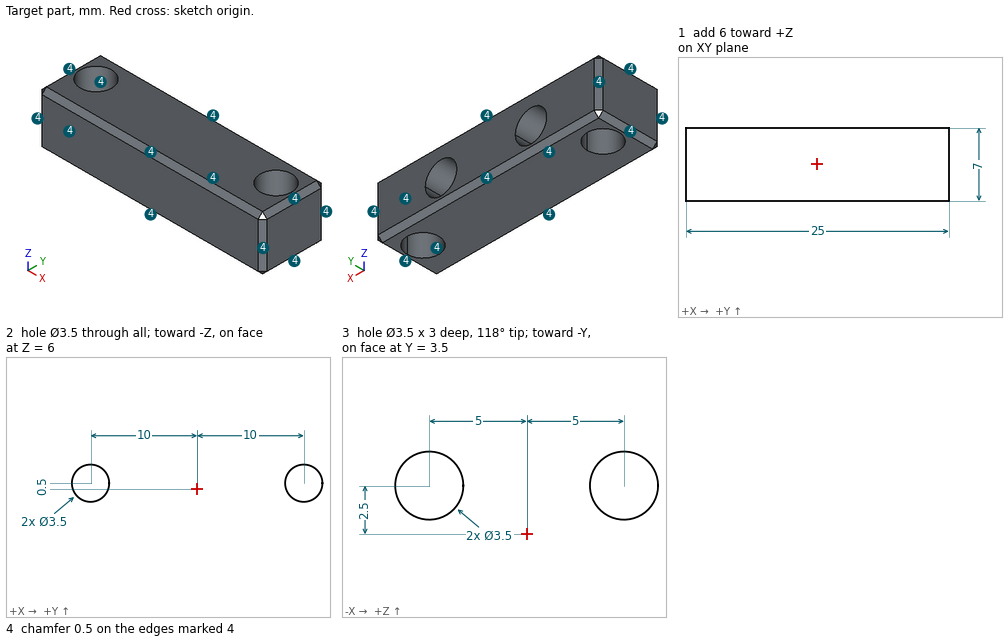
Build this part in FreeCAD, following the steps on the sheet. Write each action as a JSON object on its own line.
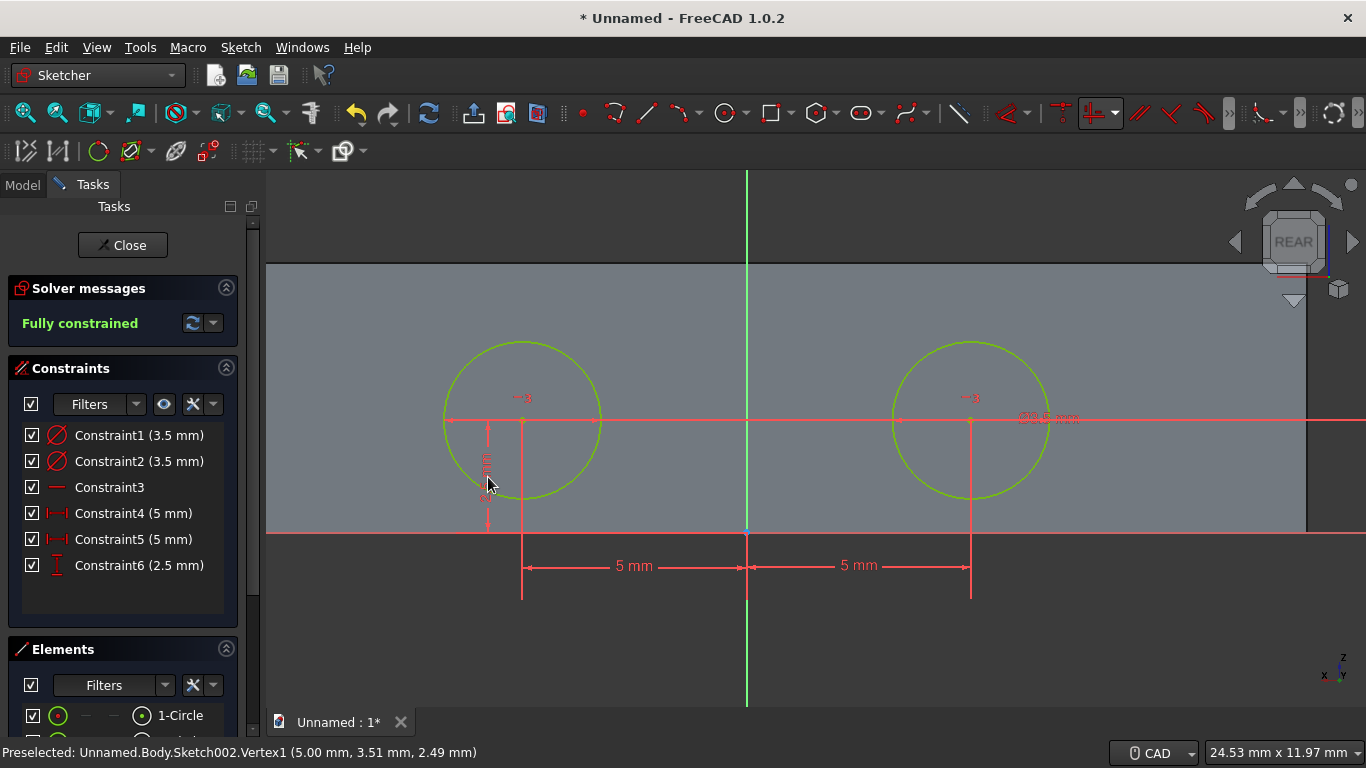
{"action": "left_click", "coordinate": [123, 245]}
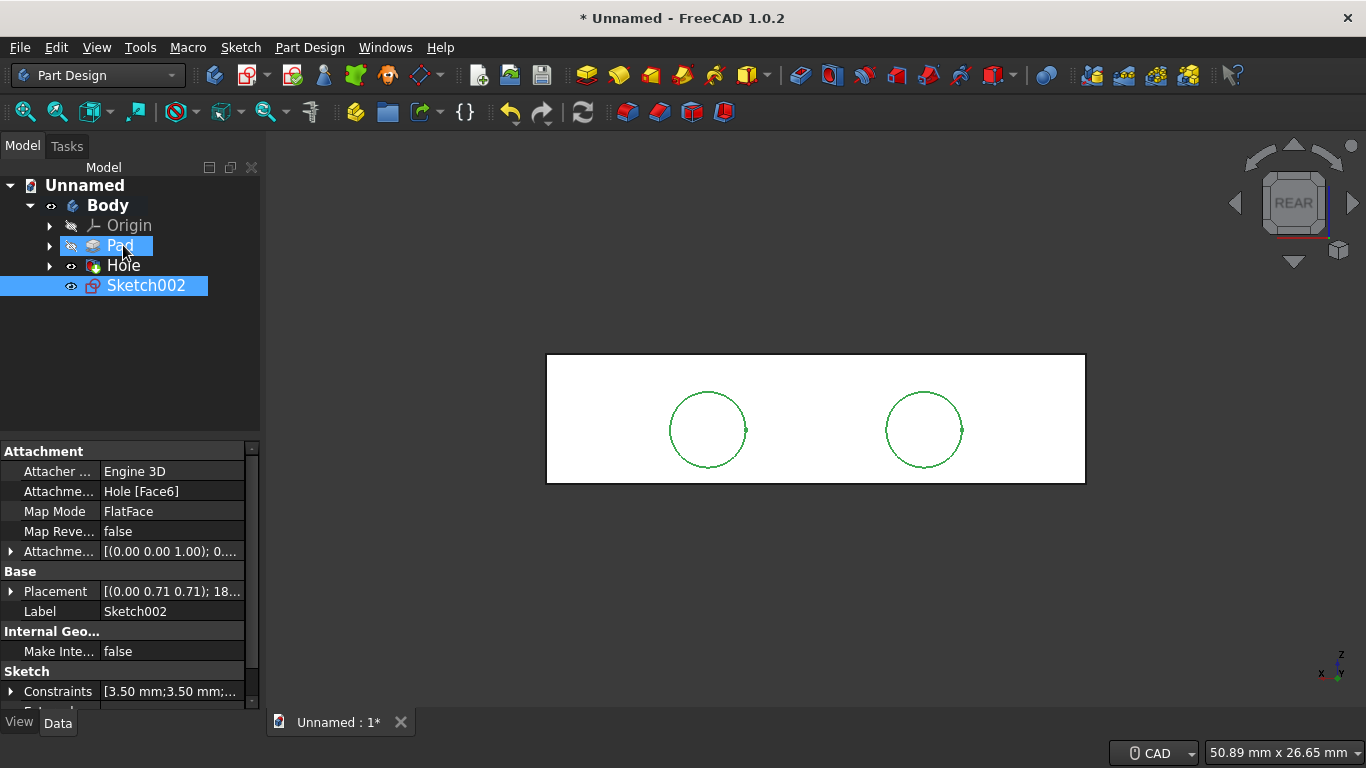
{"action": "left_click", "coordinate": [834, 76]}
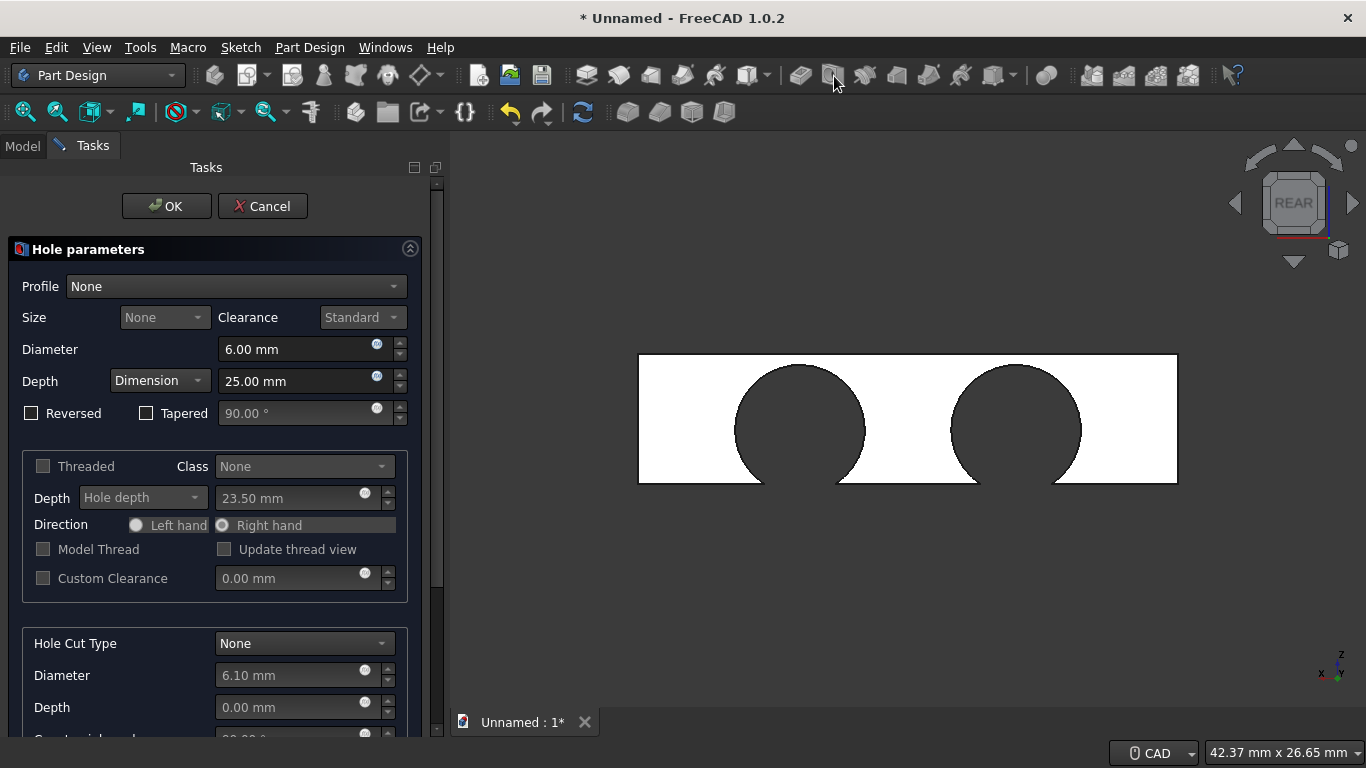
{"action": "triple_click", "coordinate": [305, 349]}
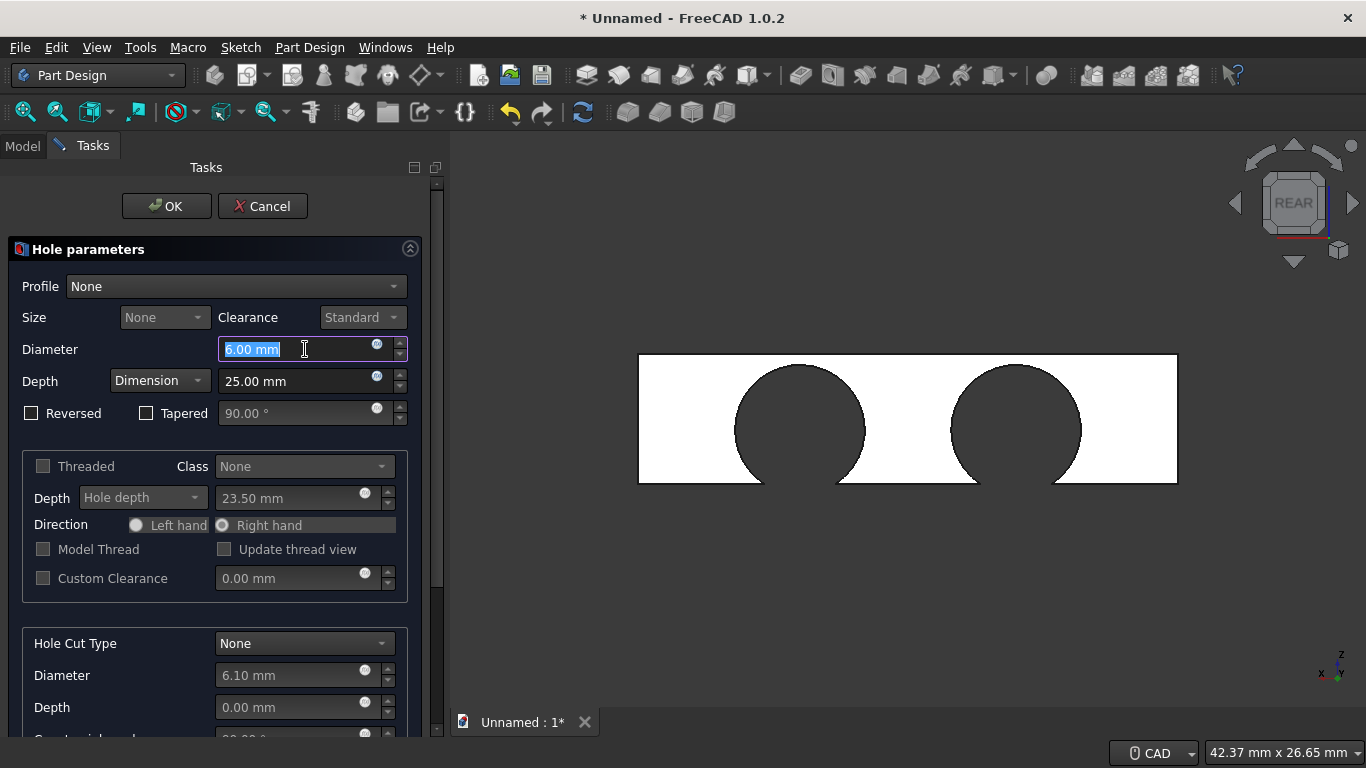
{"action": "type", "text": "3.5"}
{"action": "key", "text": "Tab"}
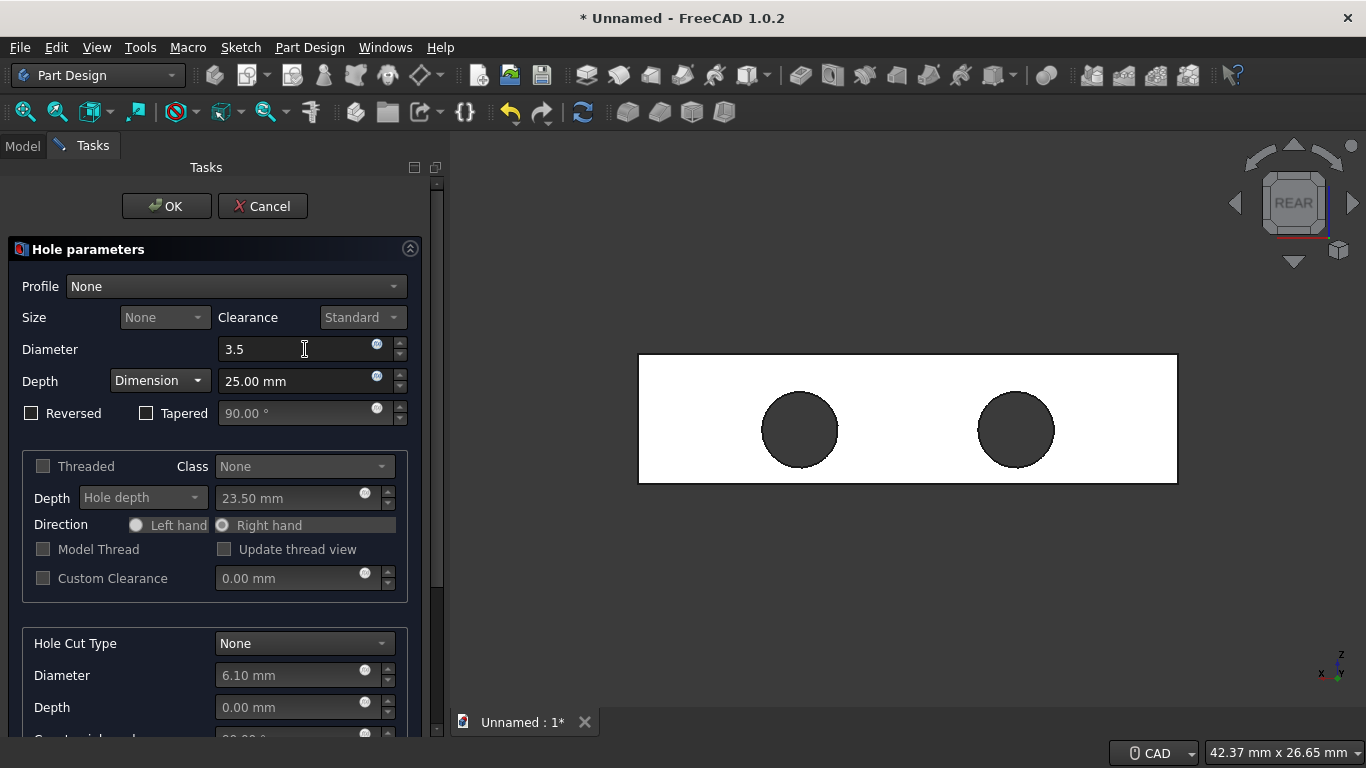
{"action": "triple_click", "coordinate": [305, 381]}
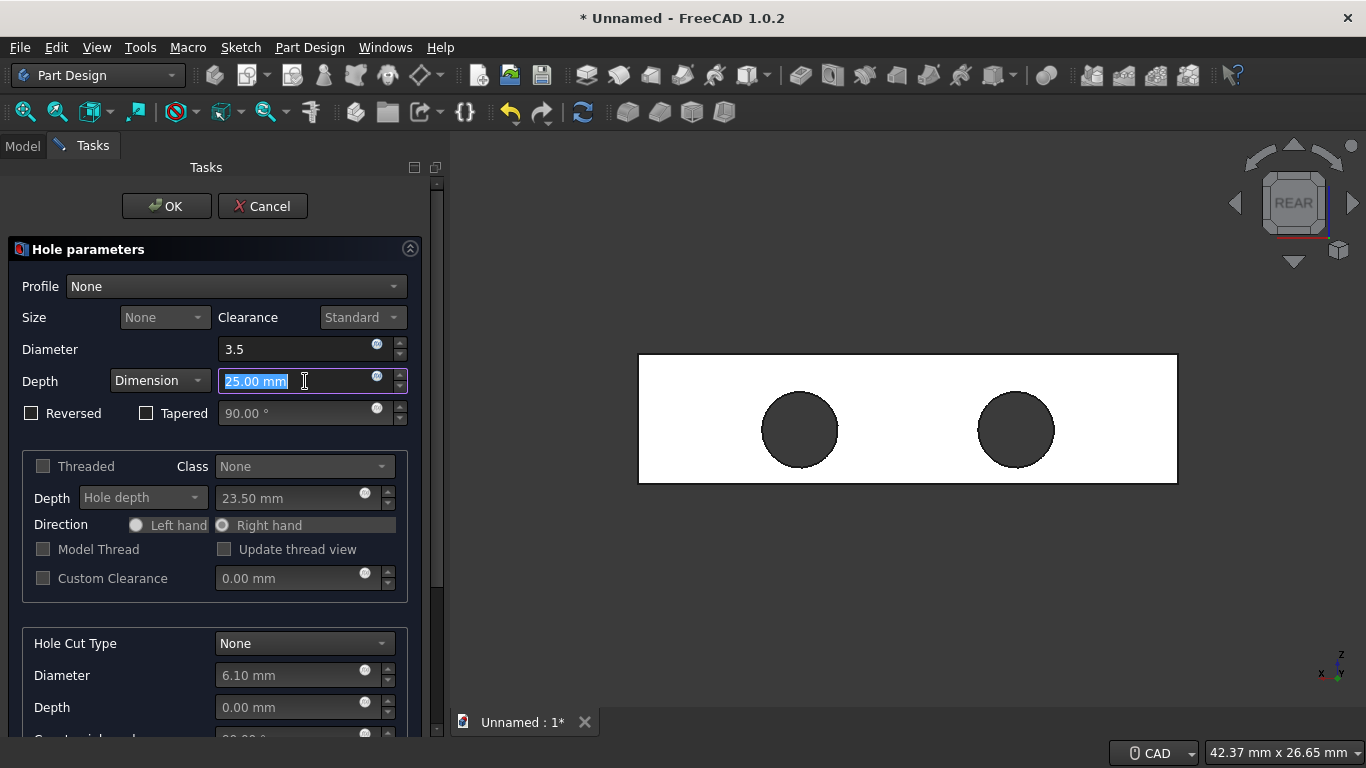
{"action": "type", "text": "3"}
{"action": "key", "text": "Tab"}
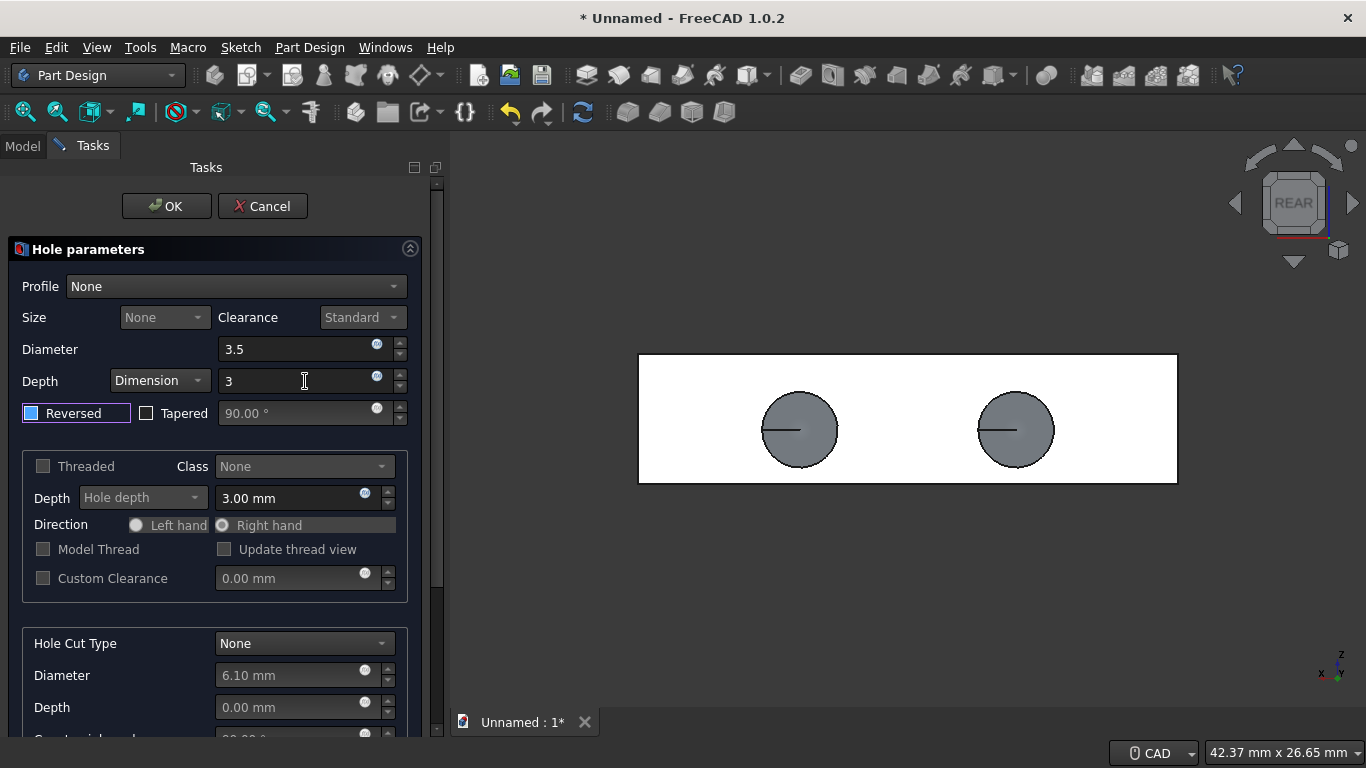
{"action": "left_click", "coordinate": [167, 206]}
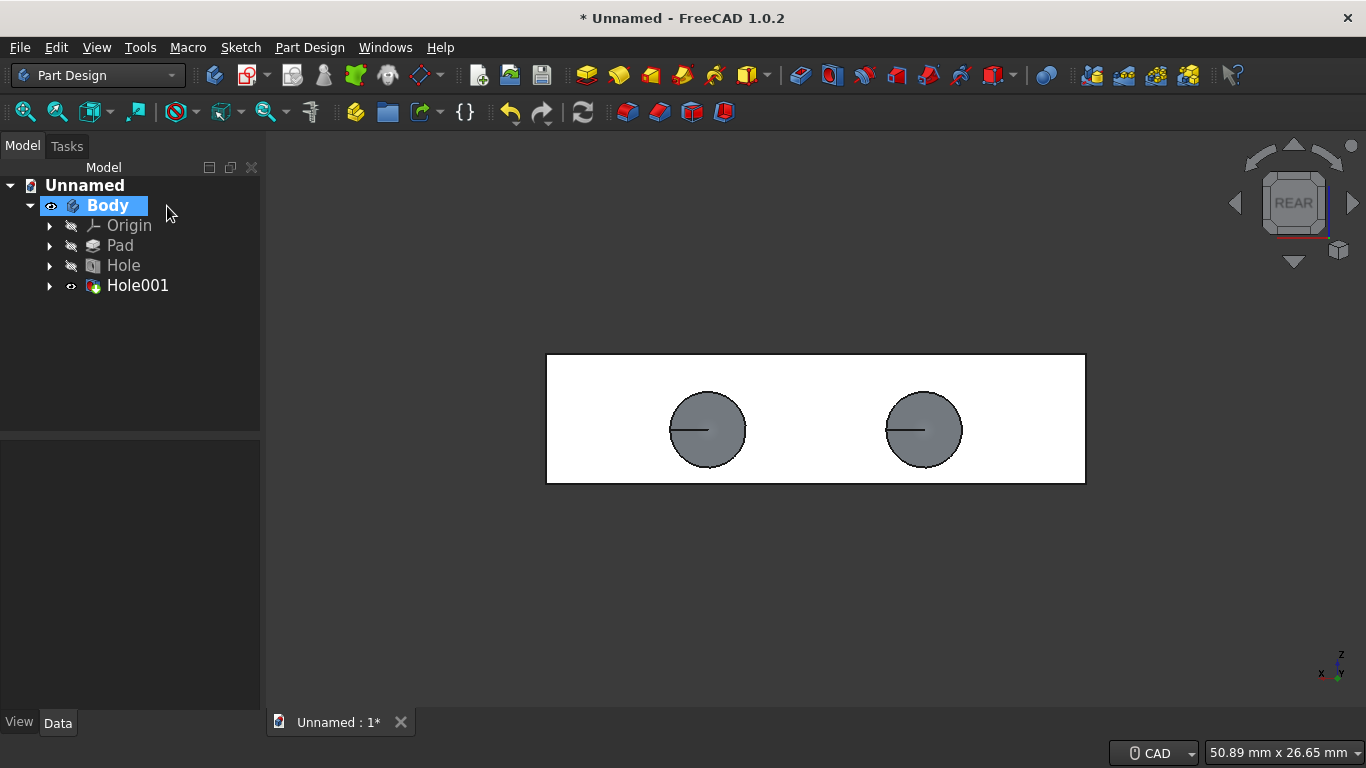
{"action": "left_click", "coordinate": [816, 483]}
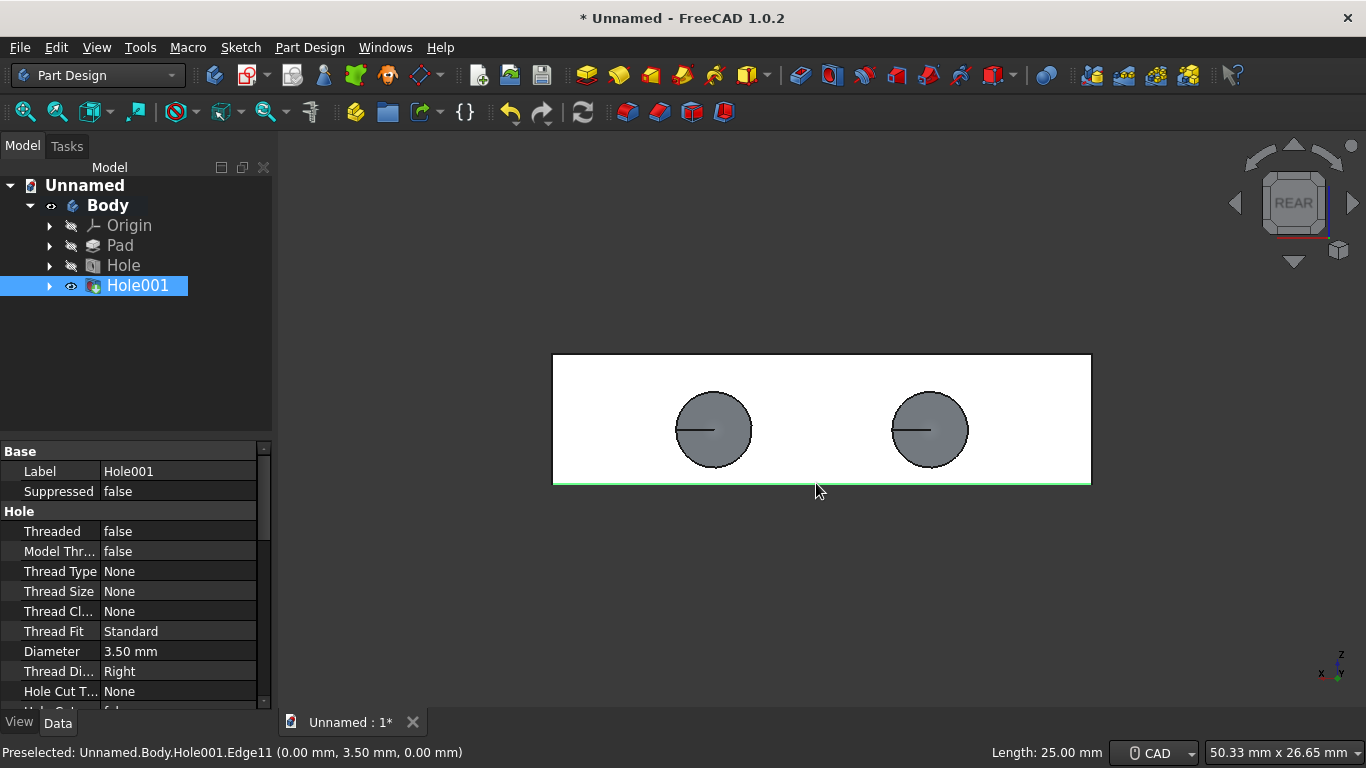
{"action": "left_click", "coordinate": [822, 353], "text": "ctrl"}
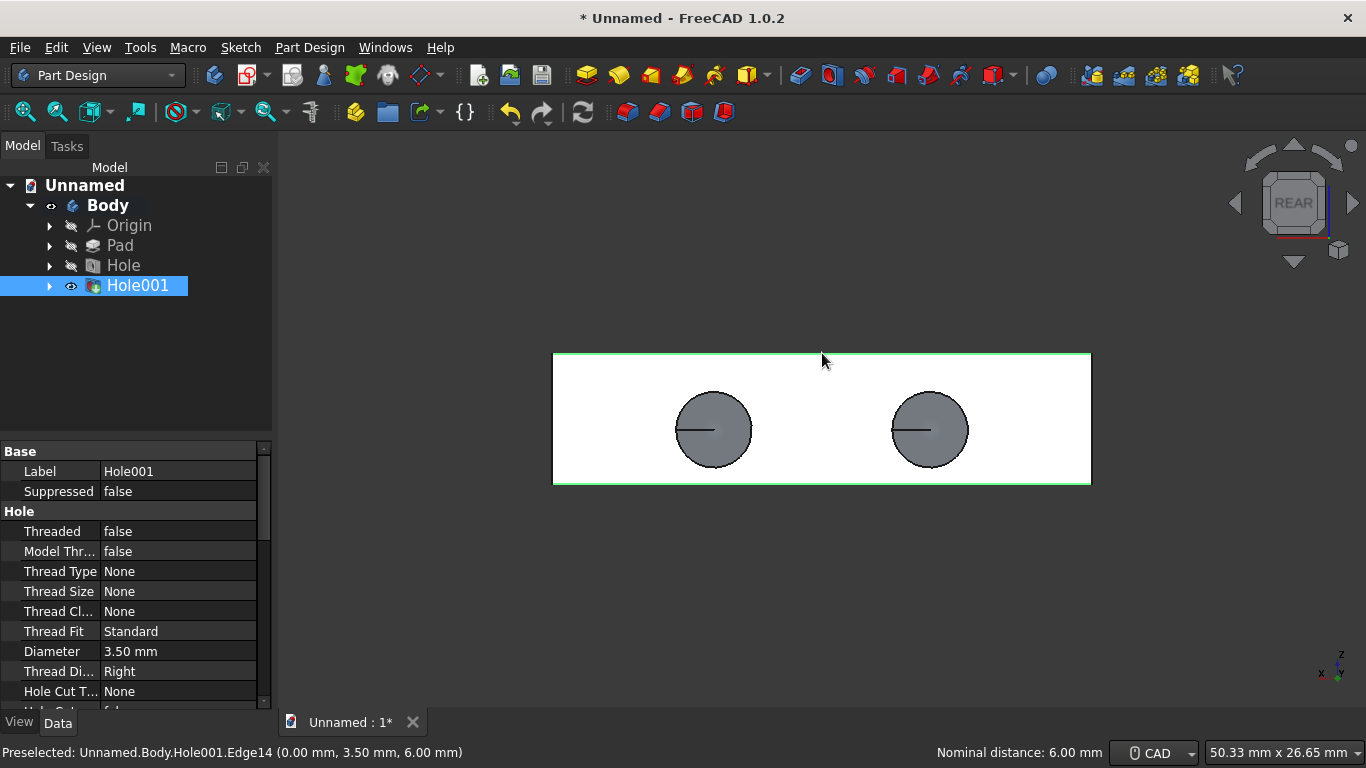
{"action": "key", "text": "0"}